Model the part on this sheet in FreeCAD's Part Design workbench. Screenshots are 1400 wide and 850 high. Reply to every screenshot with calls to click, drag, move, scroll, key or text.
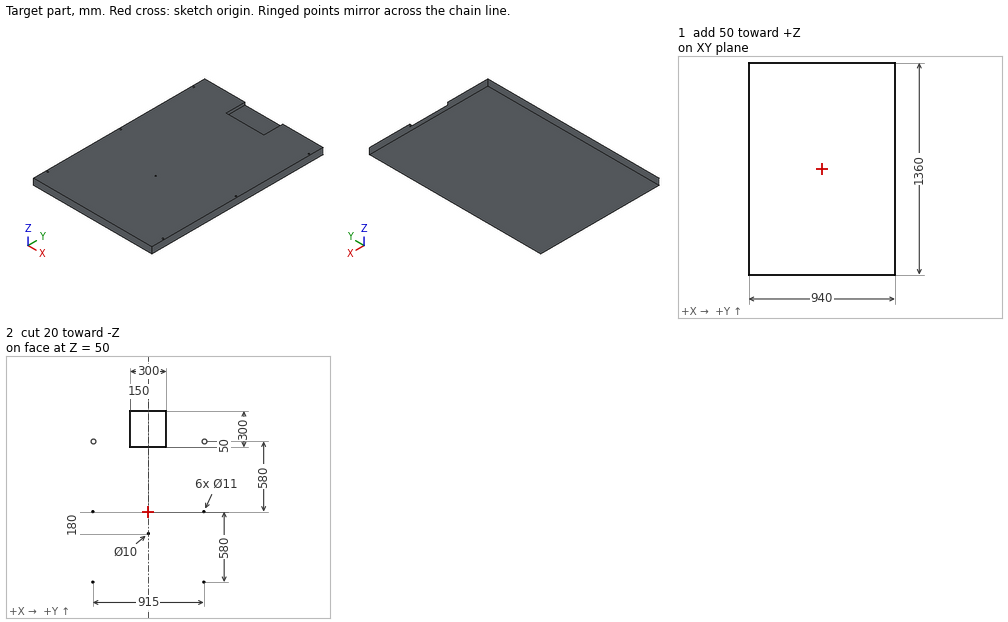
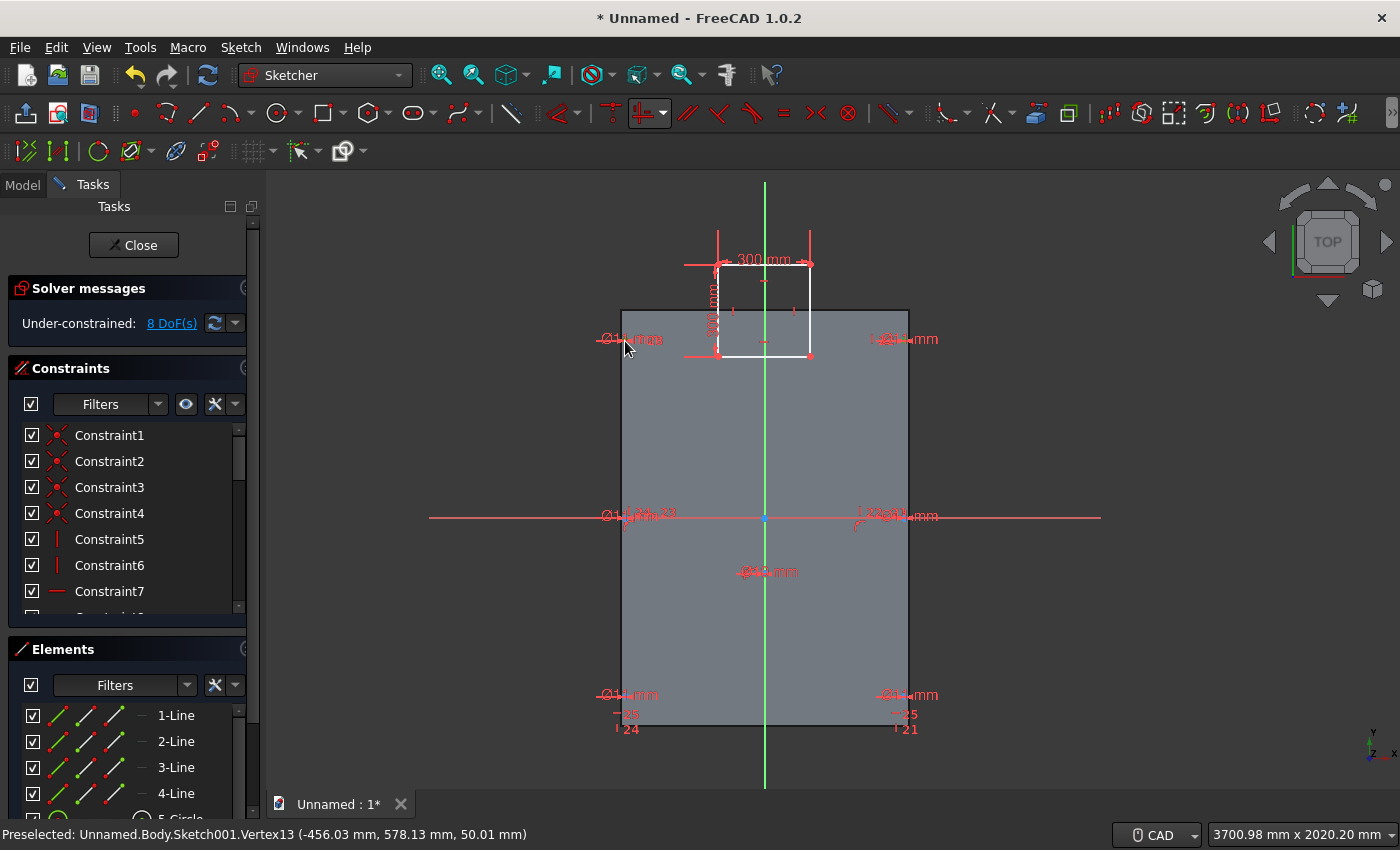
click(765, 721)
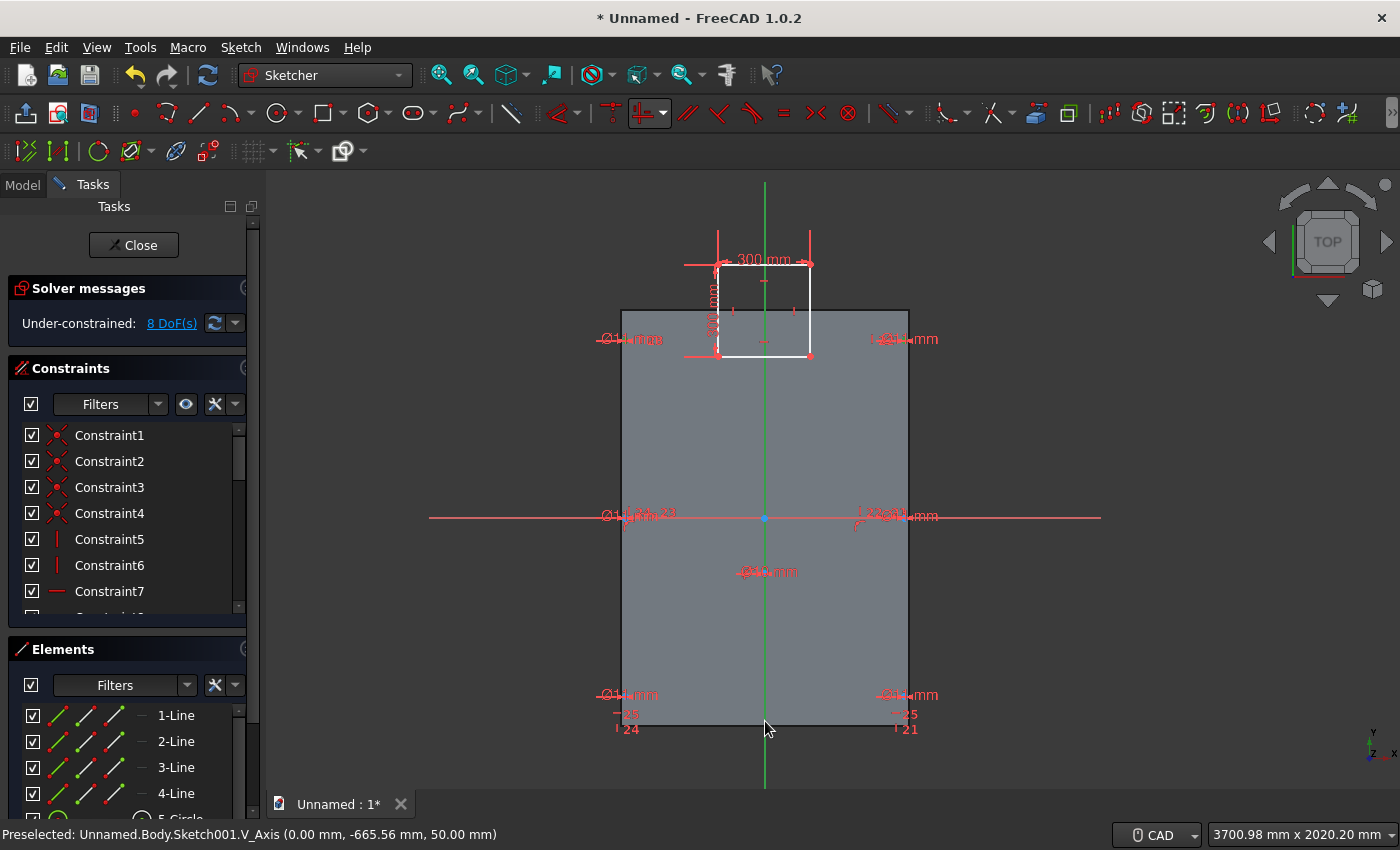
key(s)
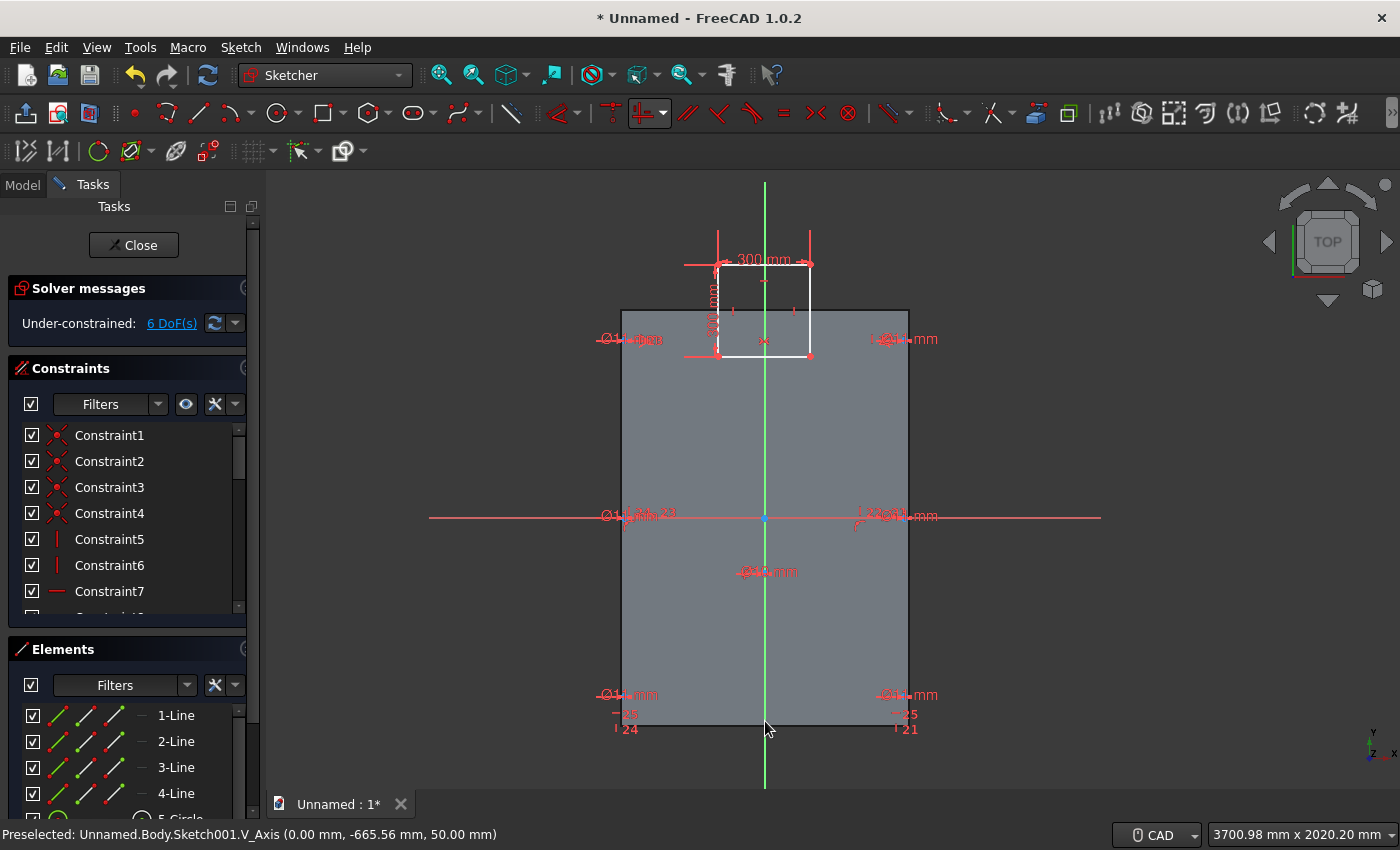
click(765, 574)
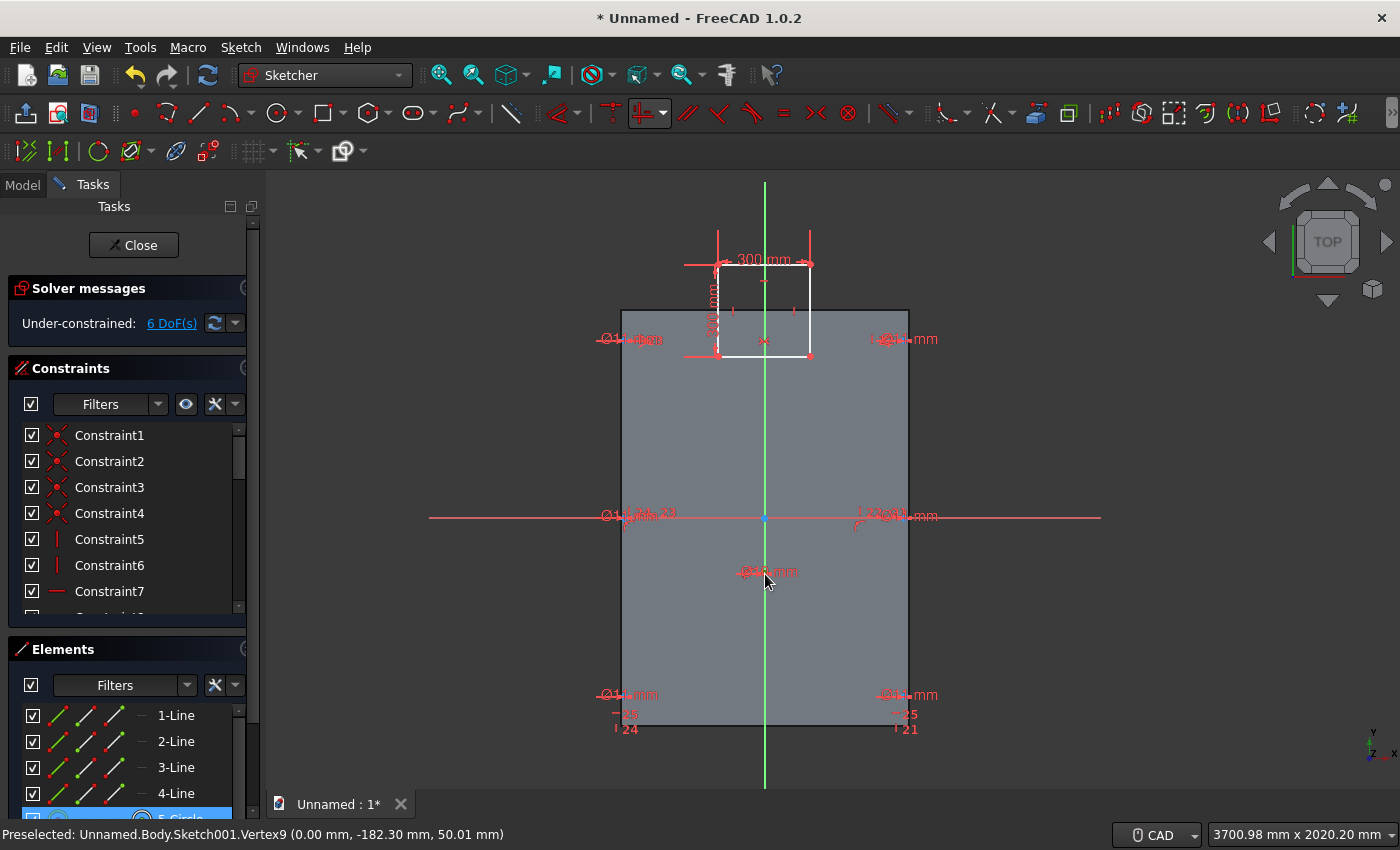
key(i)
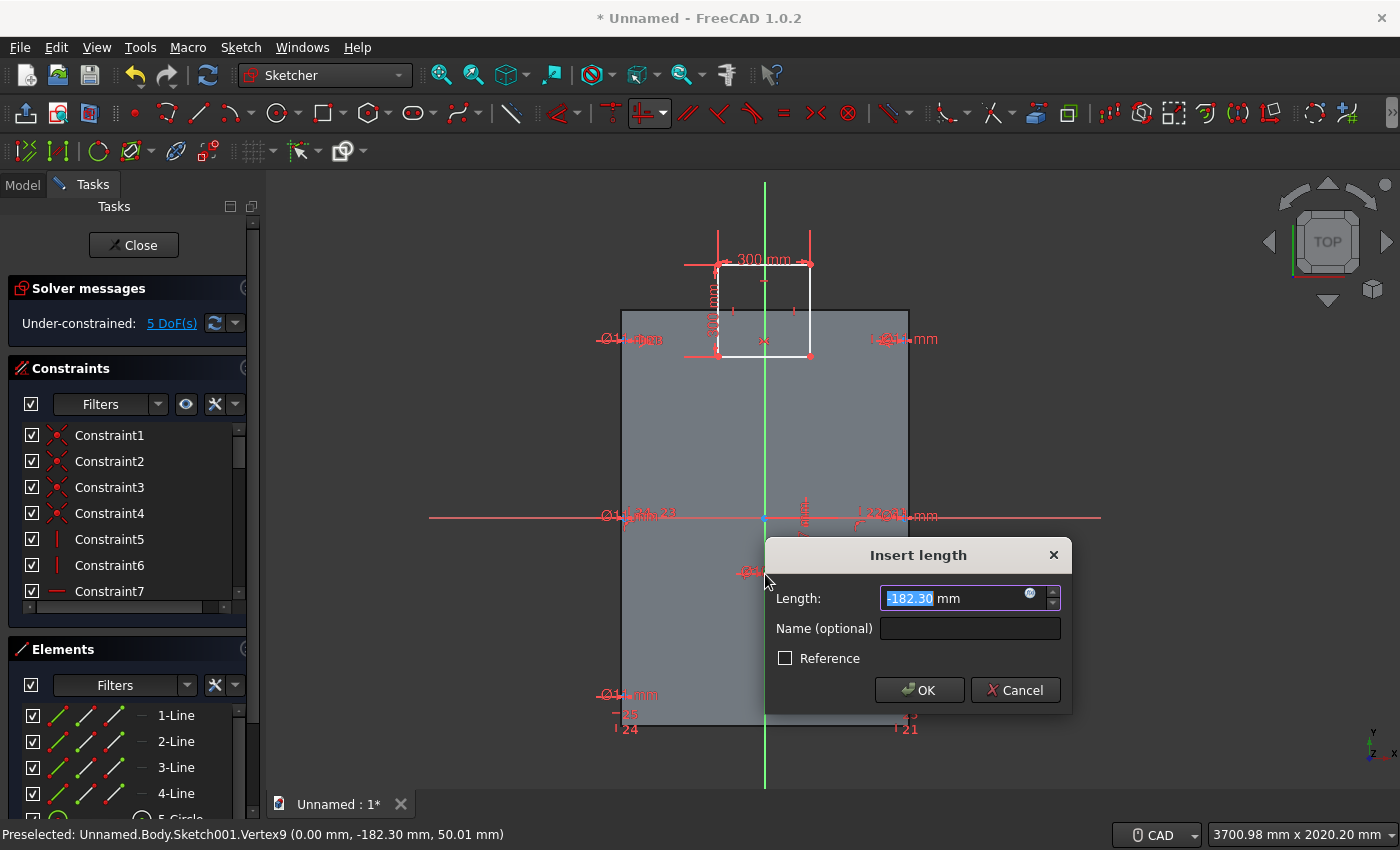
text(-180)
key(Return)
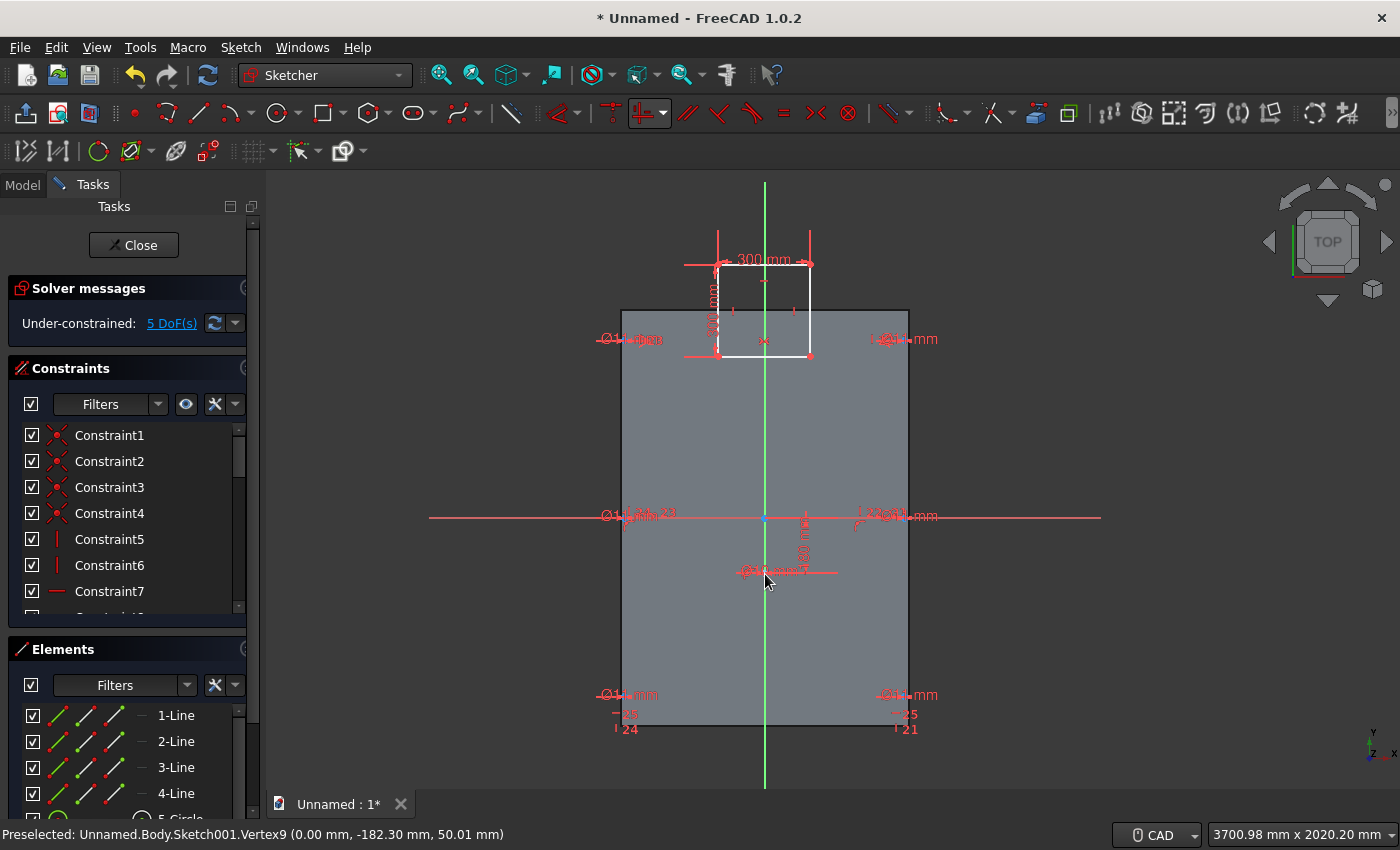
click(905, 697)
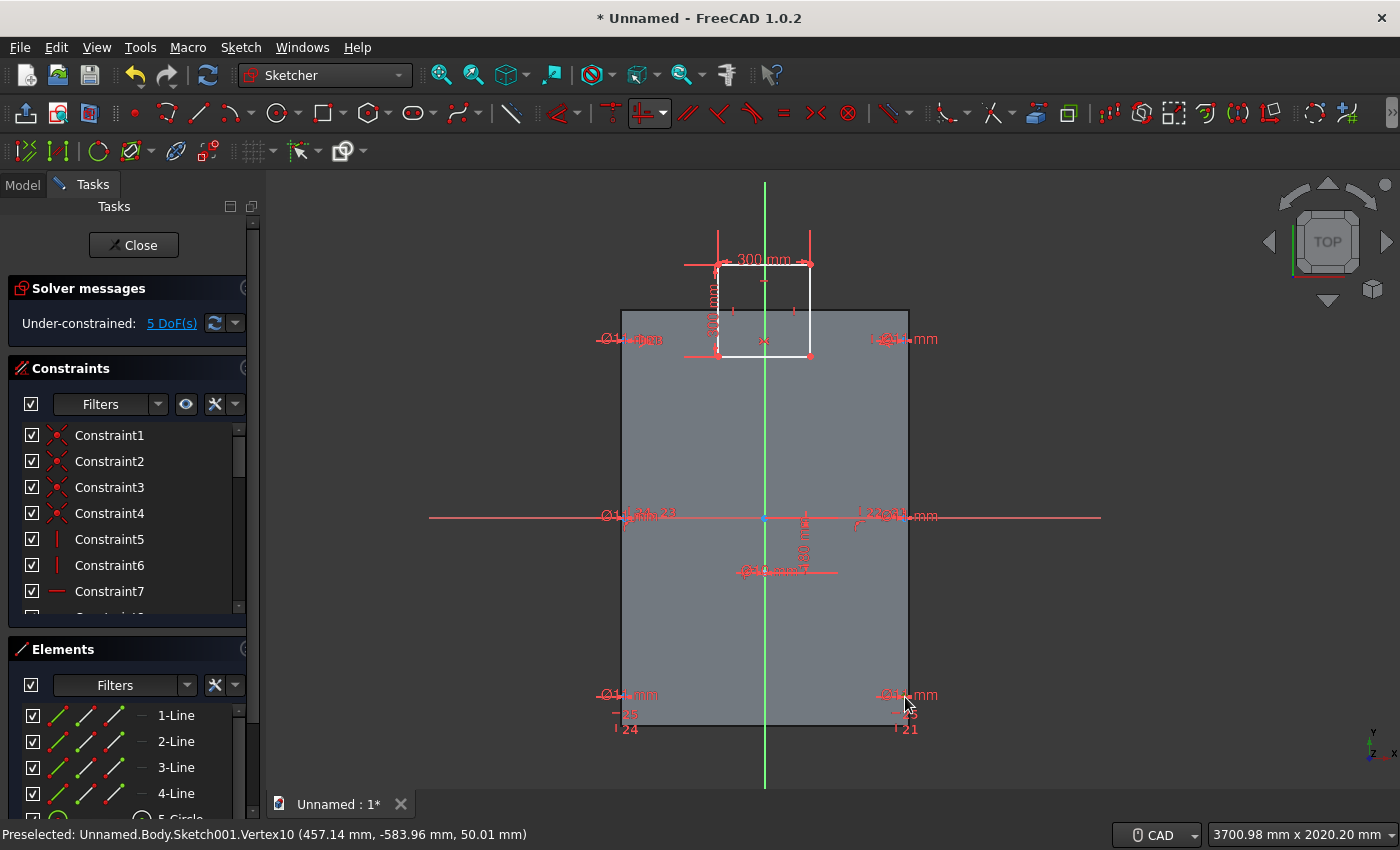
key(i)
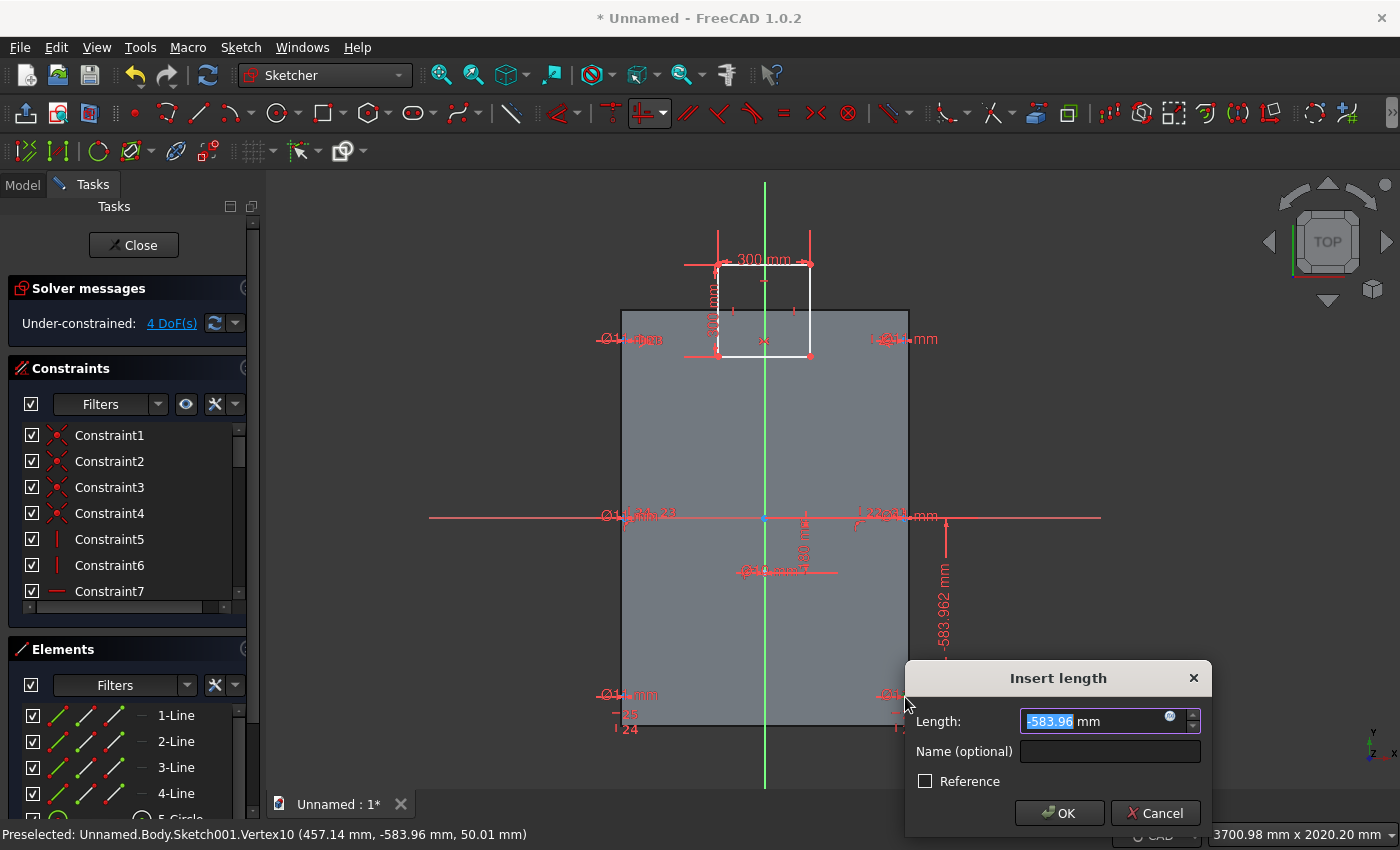
text(-580)
key(Return)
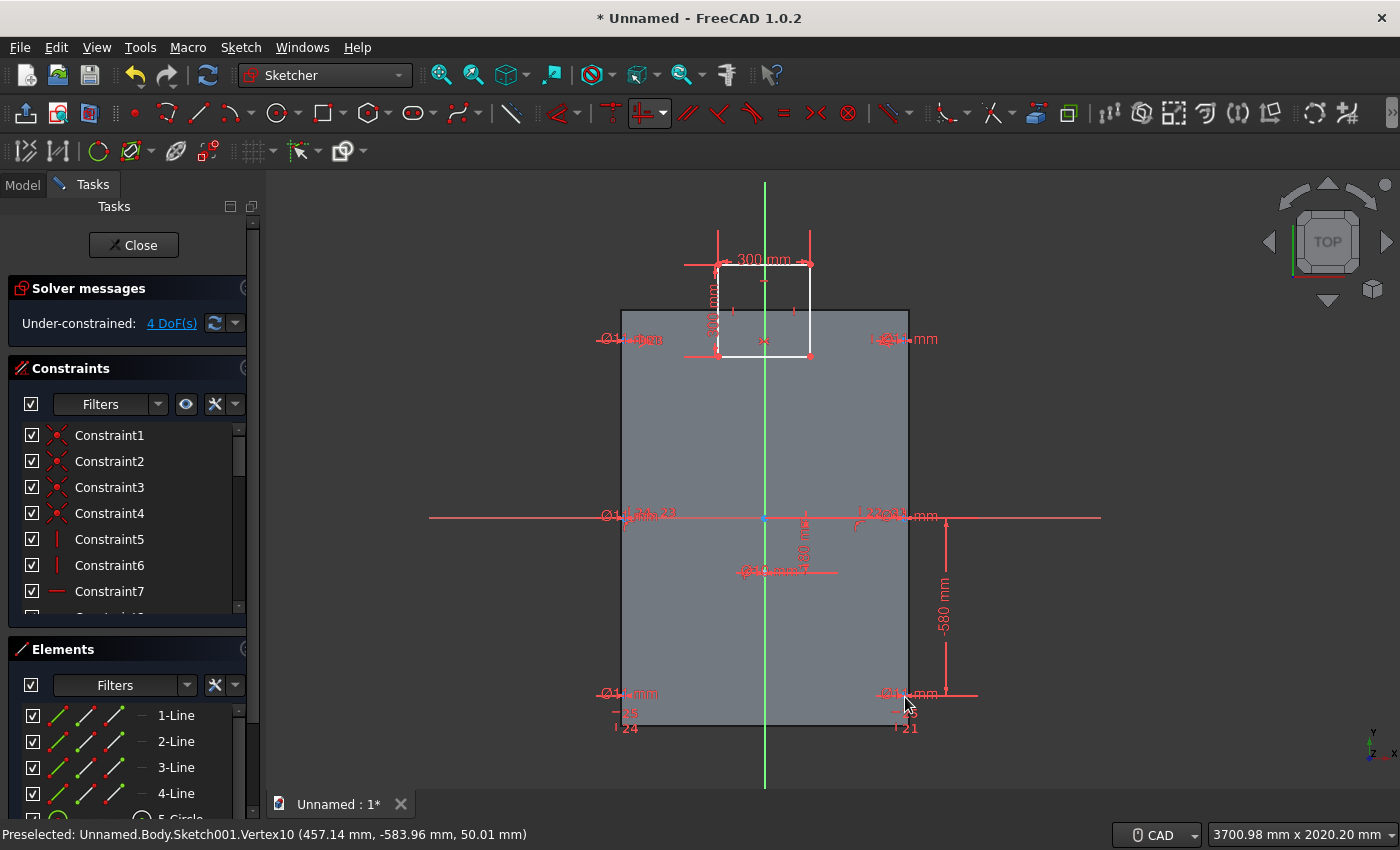
click(905, 341)